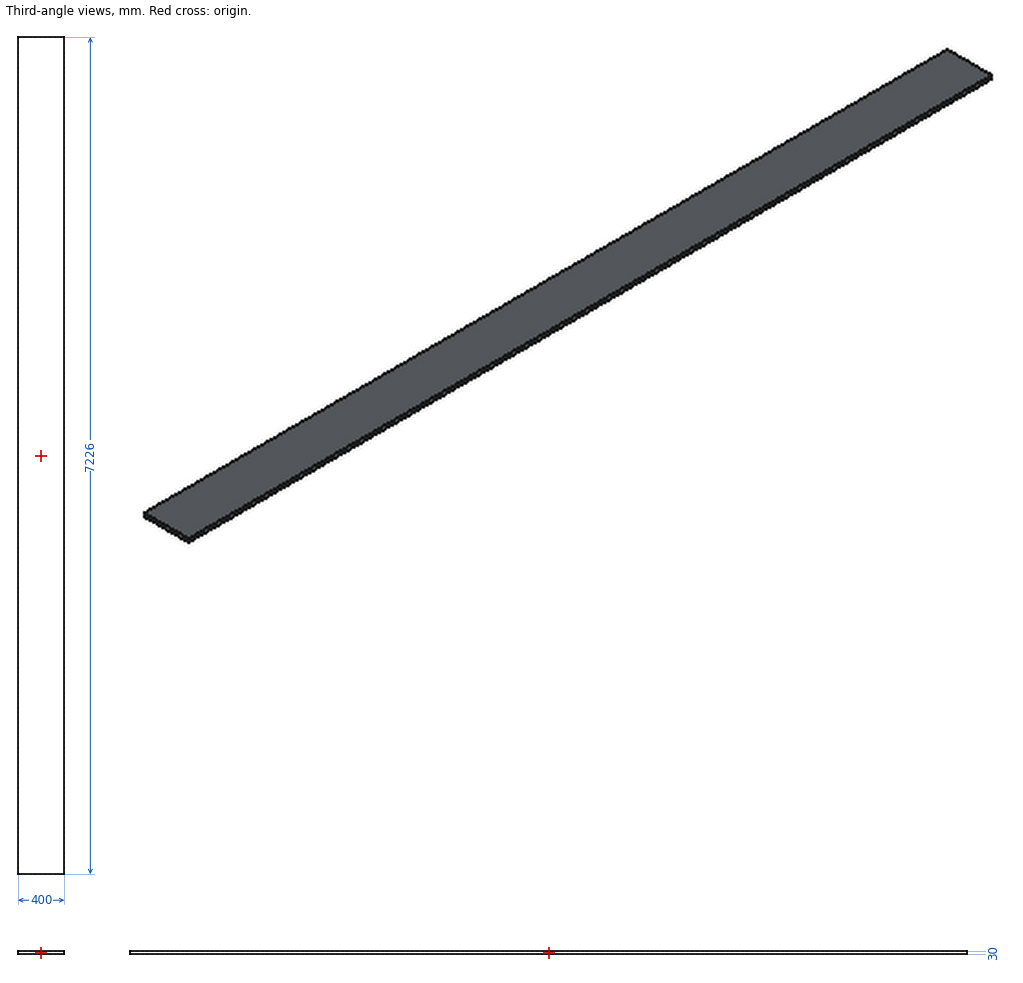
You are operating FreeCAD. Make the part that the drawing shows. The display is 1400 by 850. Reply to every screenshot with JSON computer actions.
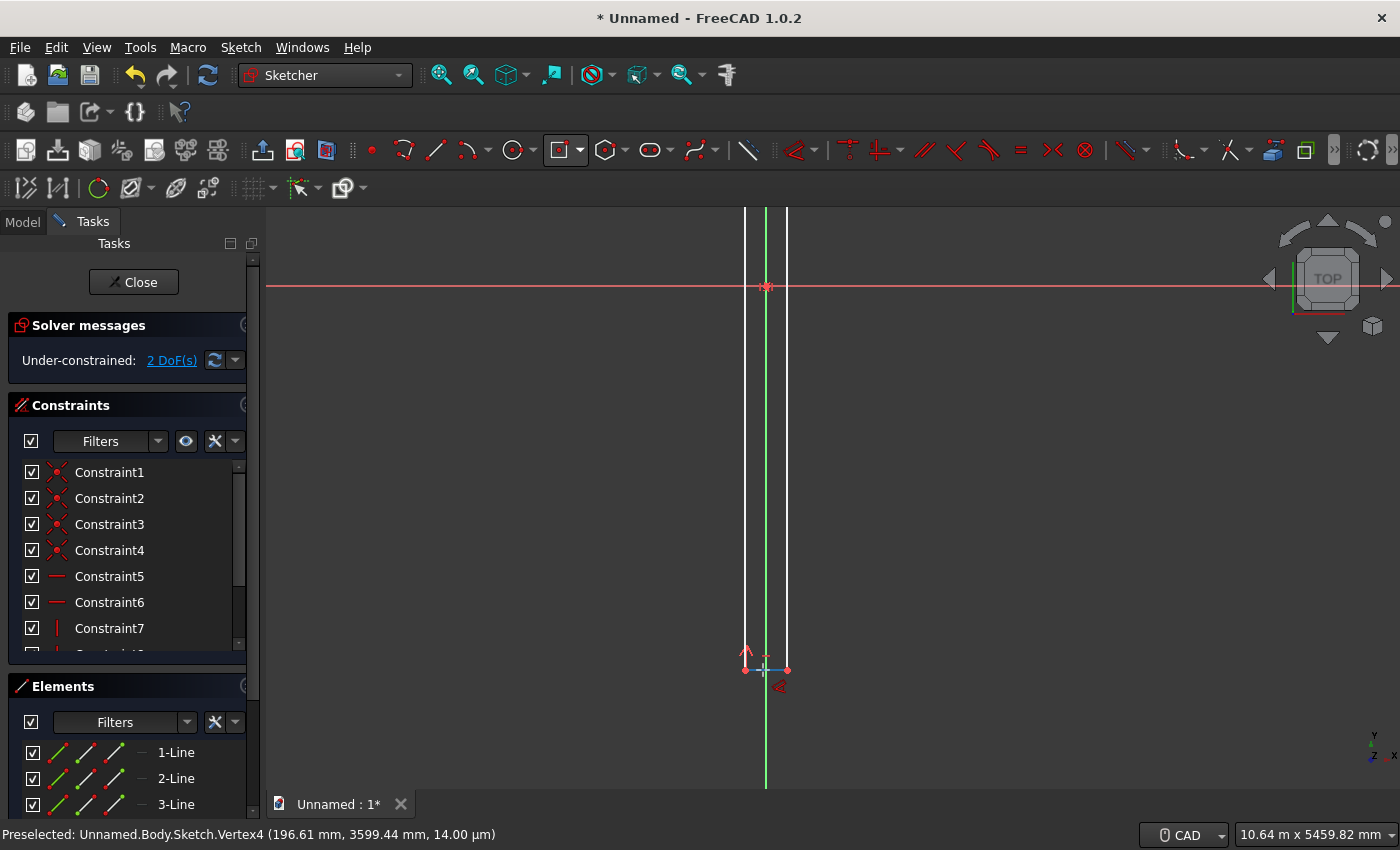
{"action": "left_click", "coordinate": [762, 670]}
{"action": "left_click", "coordinate": [752, 704]}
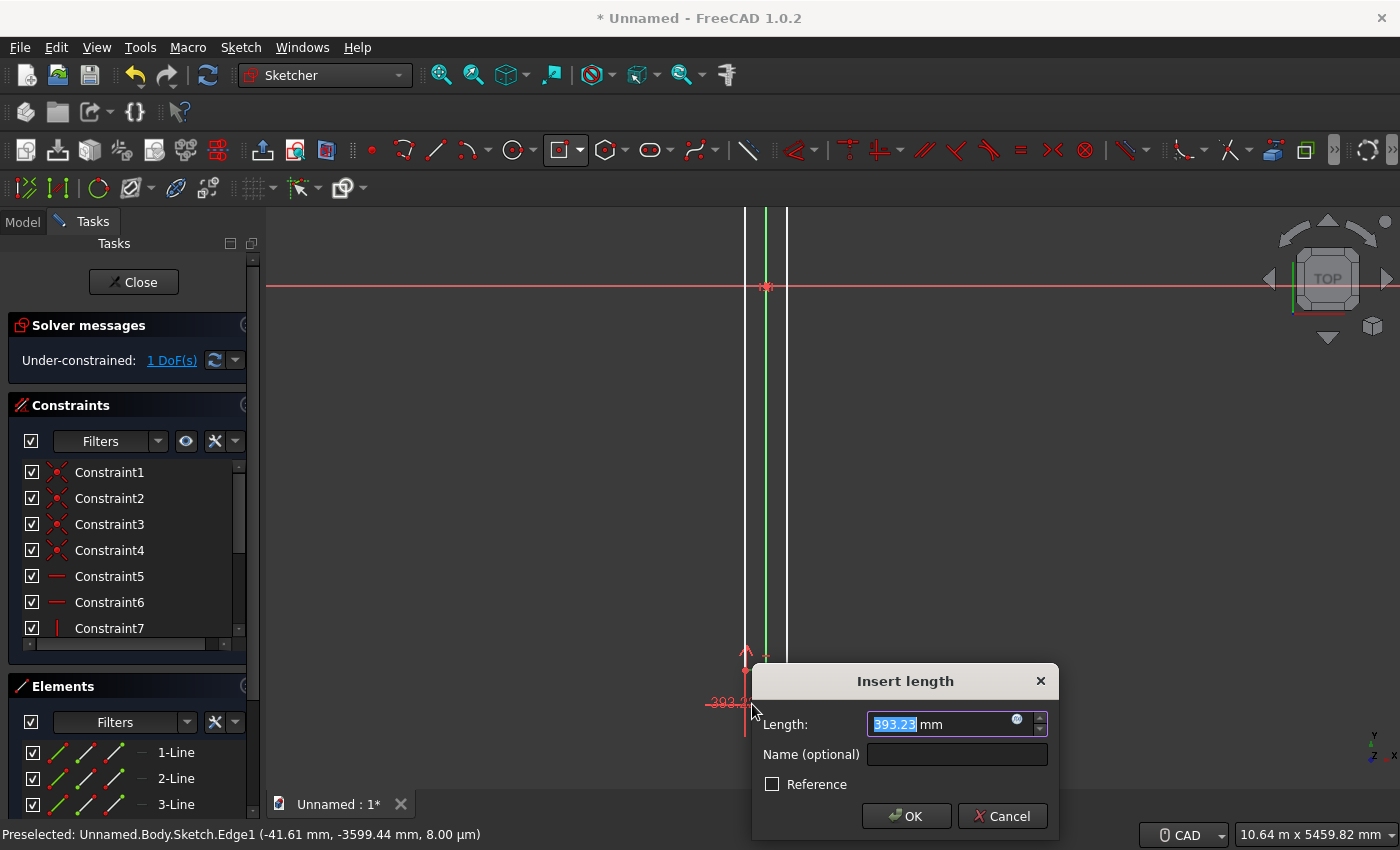
{"action": "type", "text": "400"}
{"action": "key", "text": "Return"}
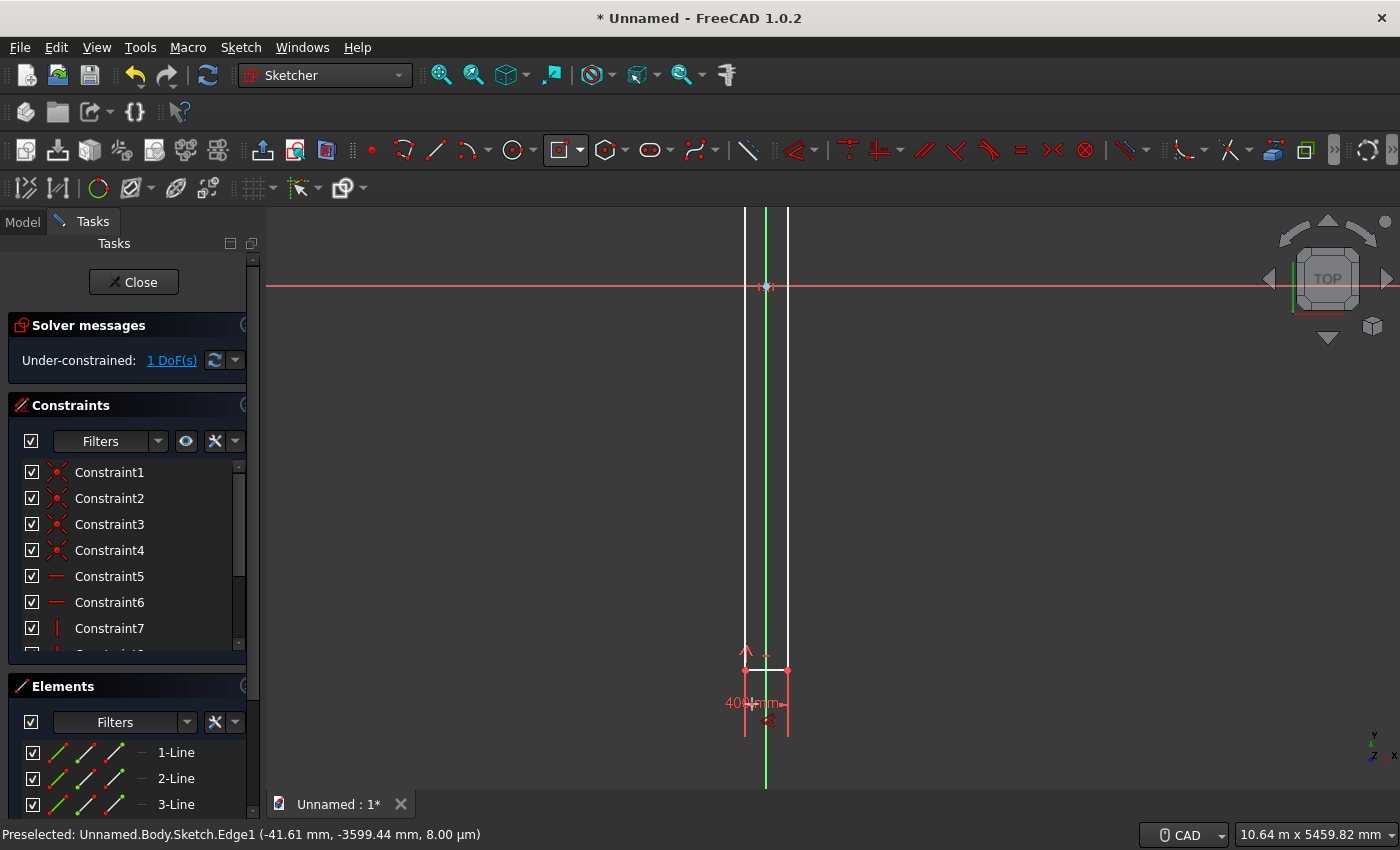
{"action": "left_click", "coordinate": [788, 440]}
{"action": "left_click", "coordinate": [822, 453]}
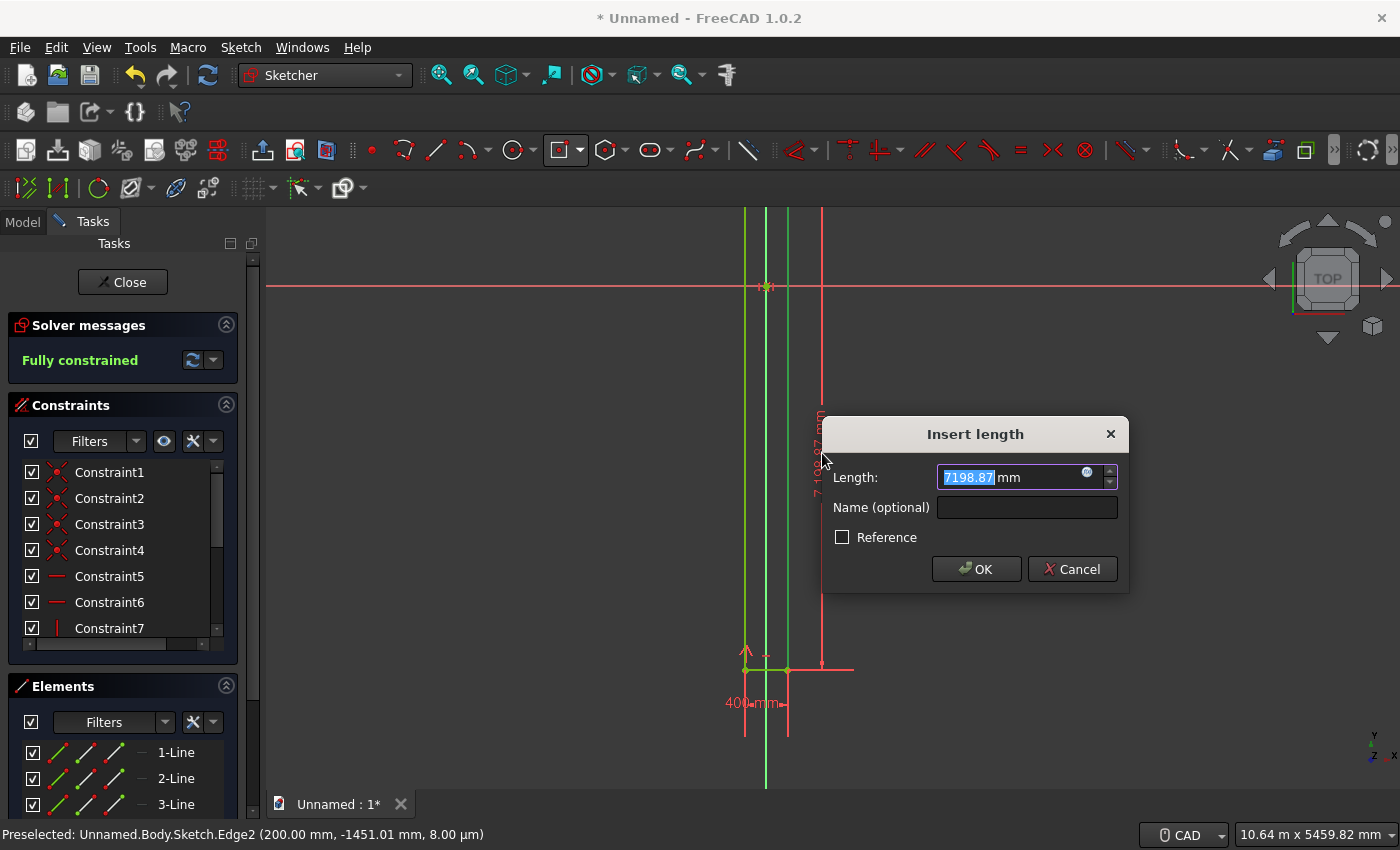
{"action": "type", "text": "7226"}
{"action": "key", "text": "Return"}
{"action": "key", "text": "Escape"}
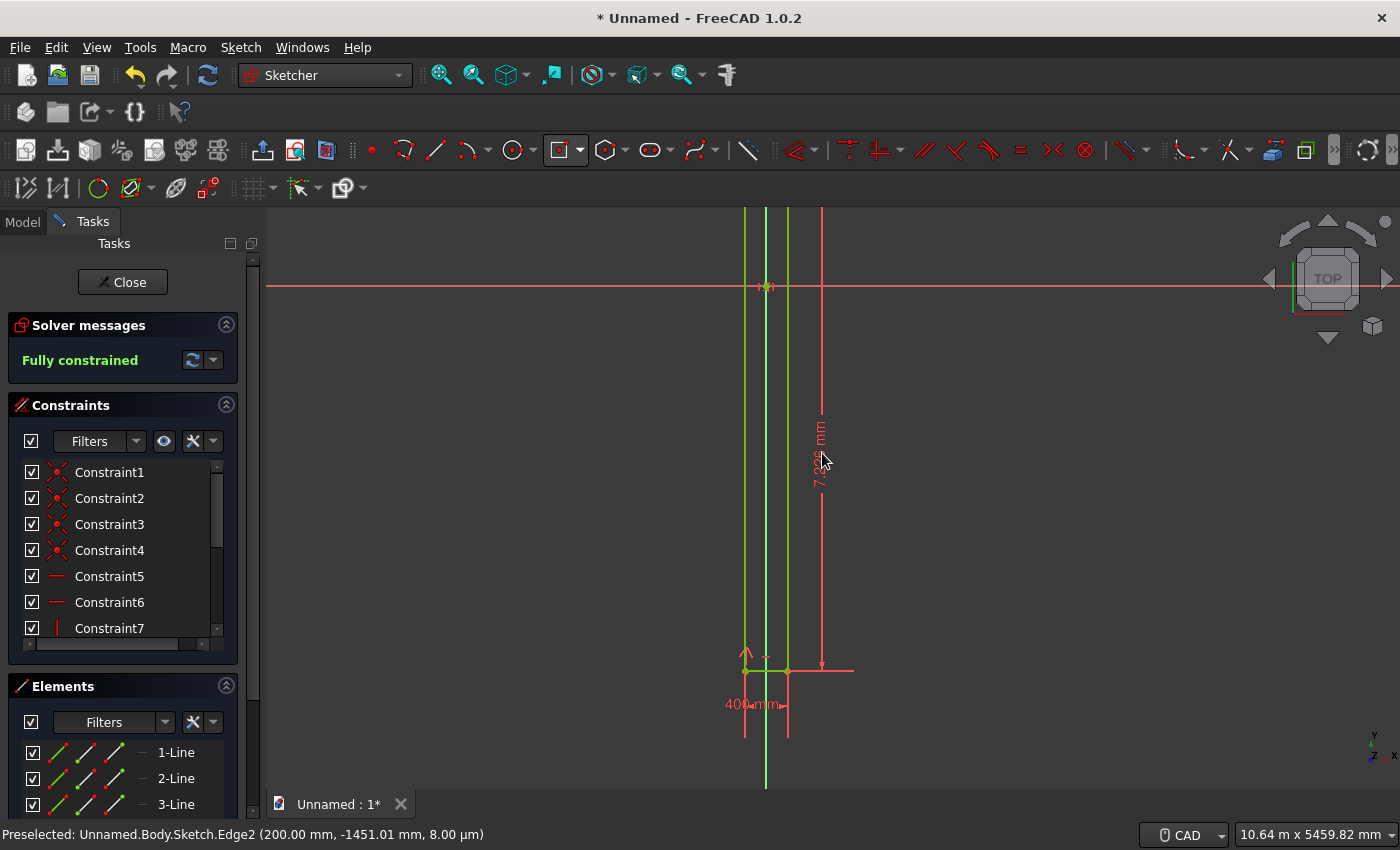
{"action": "left_click", "coordinate": [123, 282]}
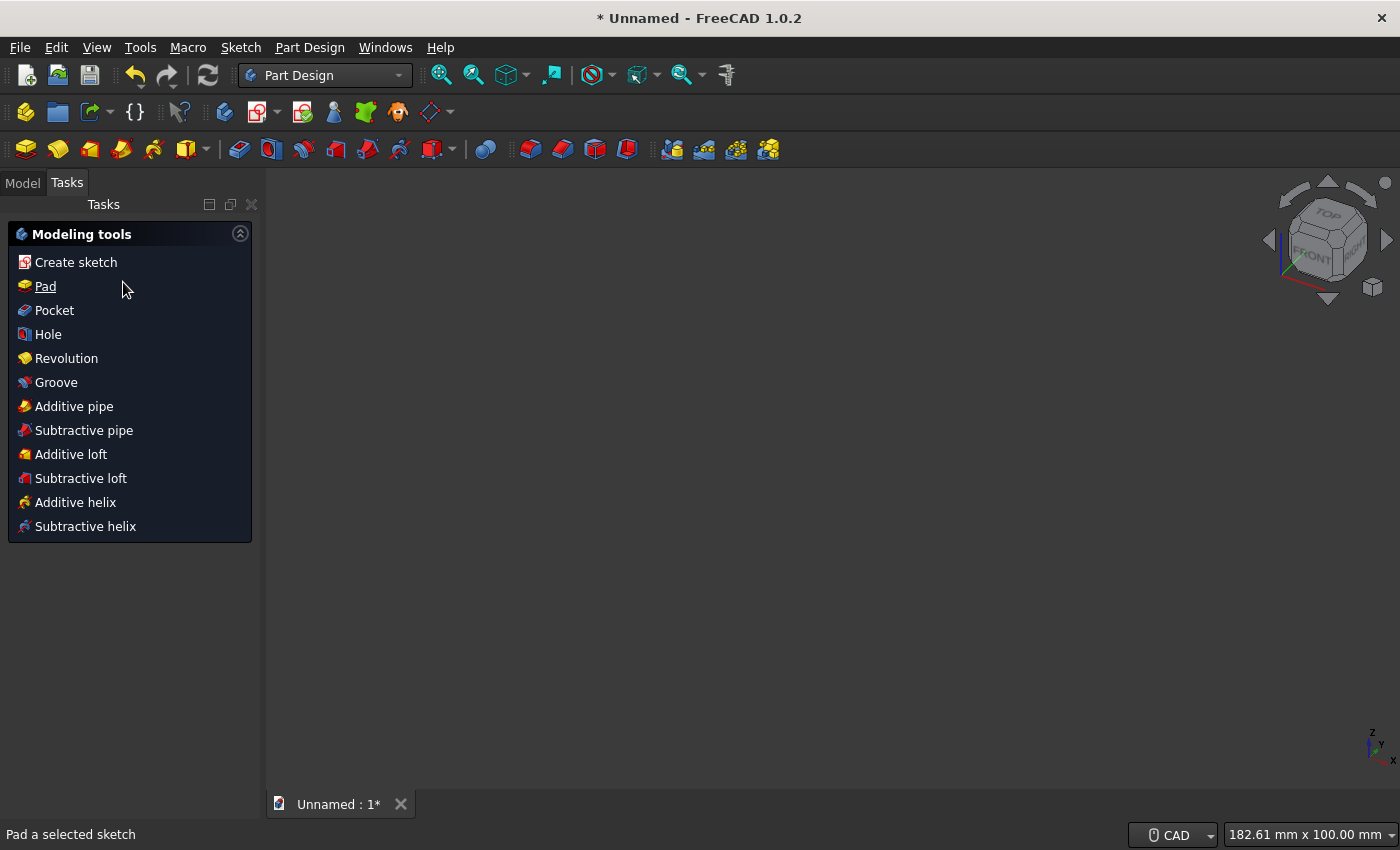
{"action": "left_click", "coordinate": [26, 150]}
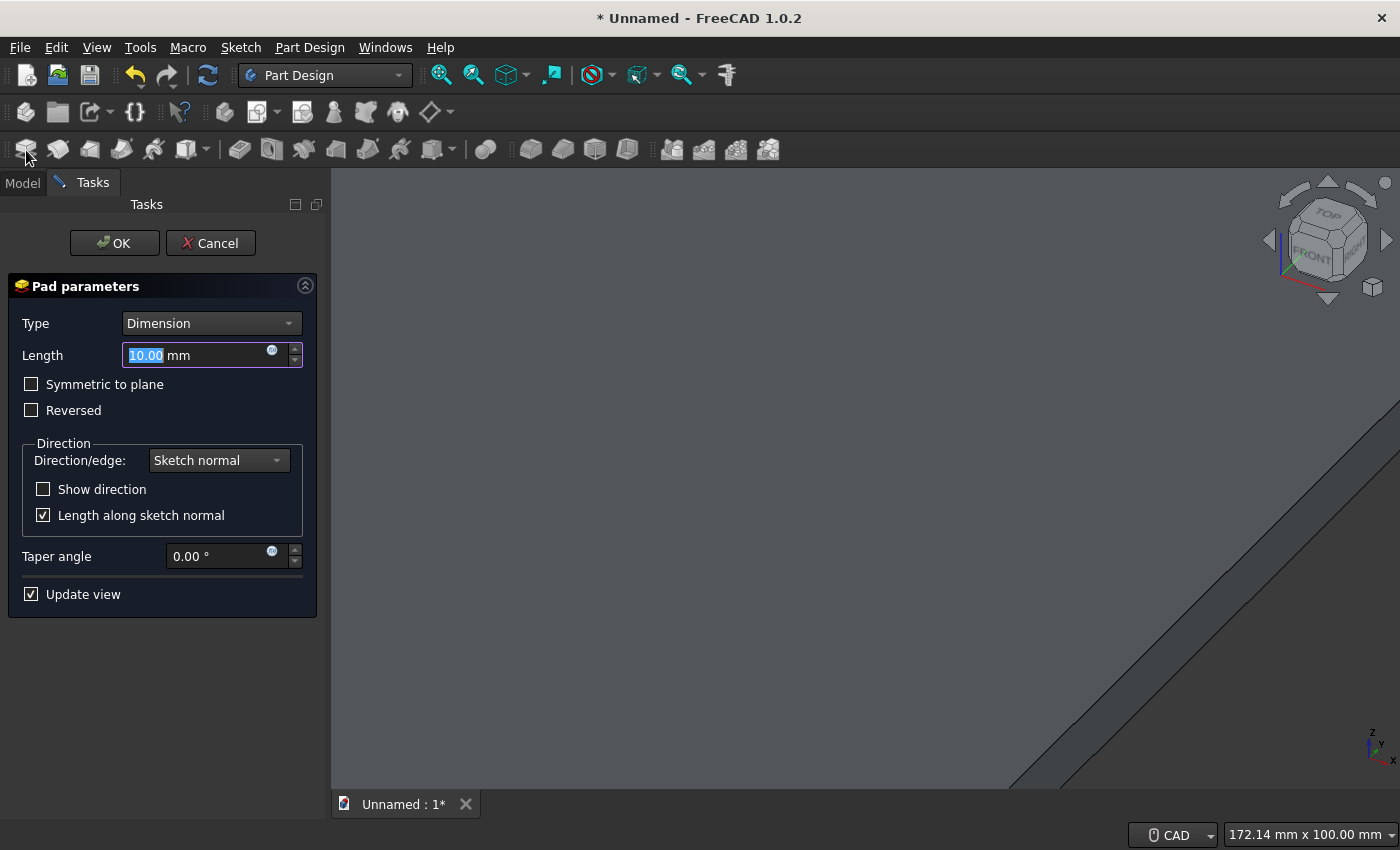
{"action": "type", "text": "30"}
{"action": "key", "text": "Tab"}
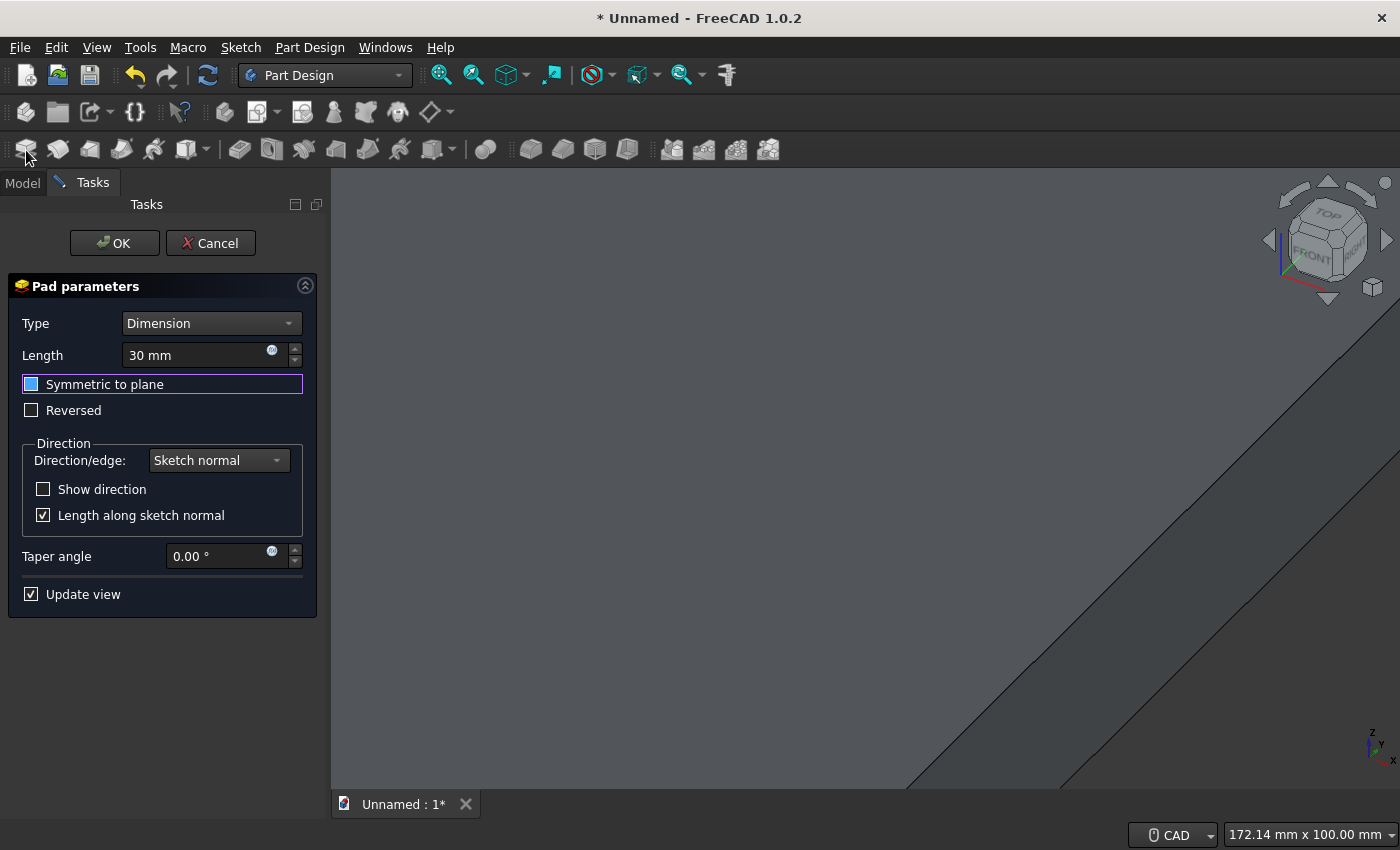
{"action": "left_click", "coordinate": [30, 384]}